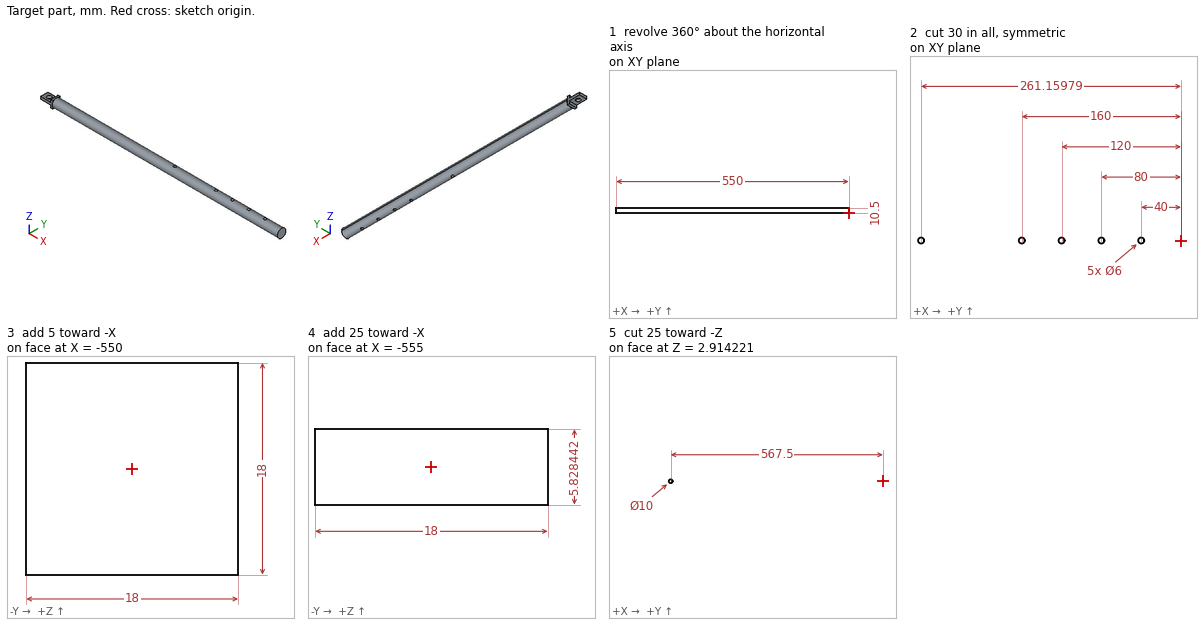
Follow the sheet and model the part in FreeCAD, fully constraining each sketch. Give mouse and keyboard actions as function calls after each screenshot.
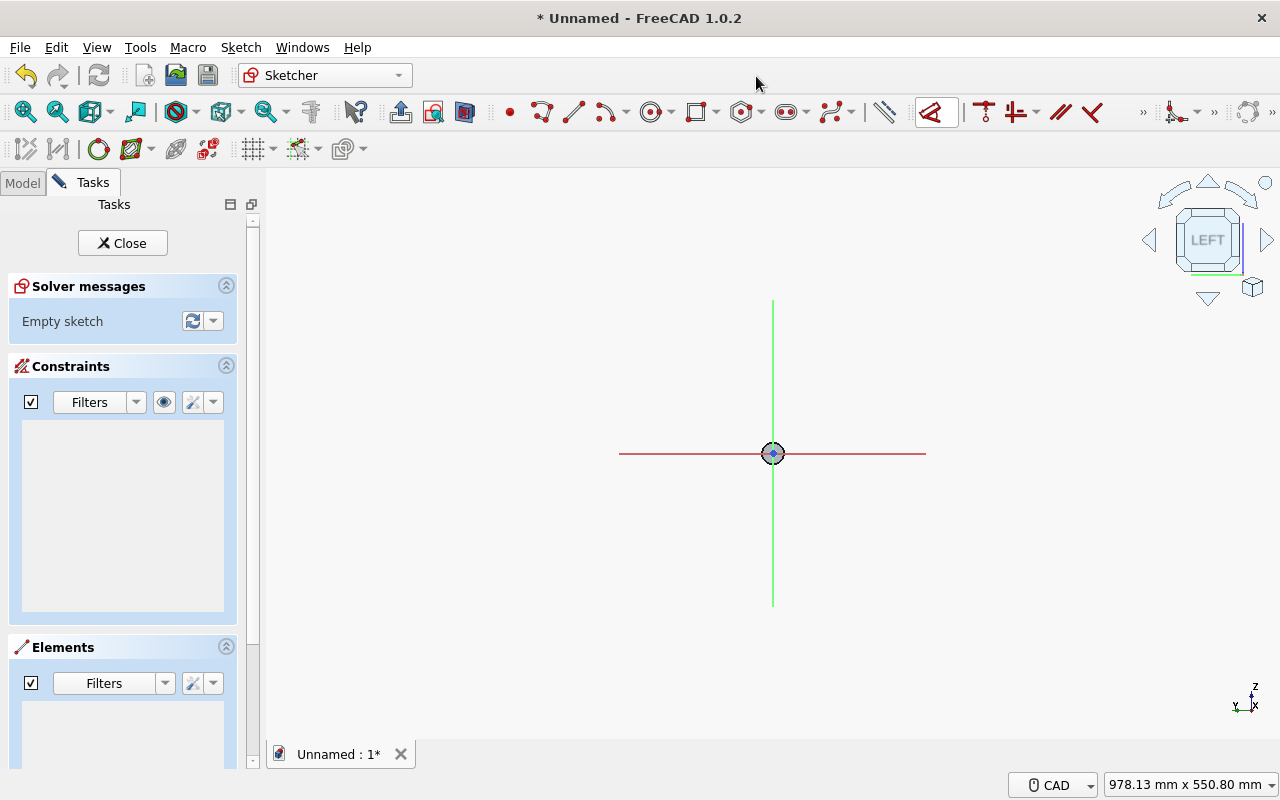
scroll(777, 454, up, 15)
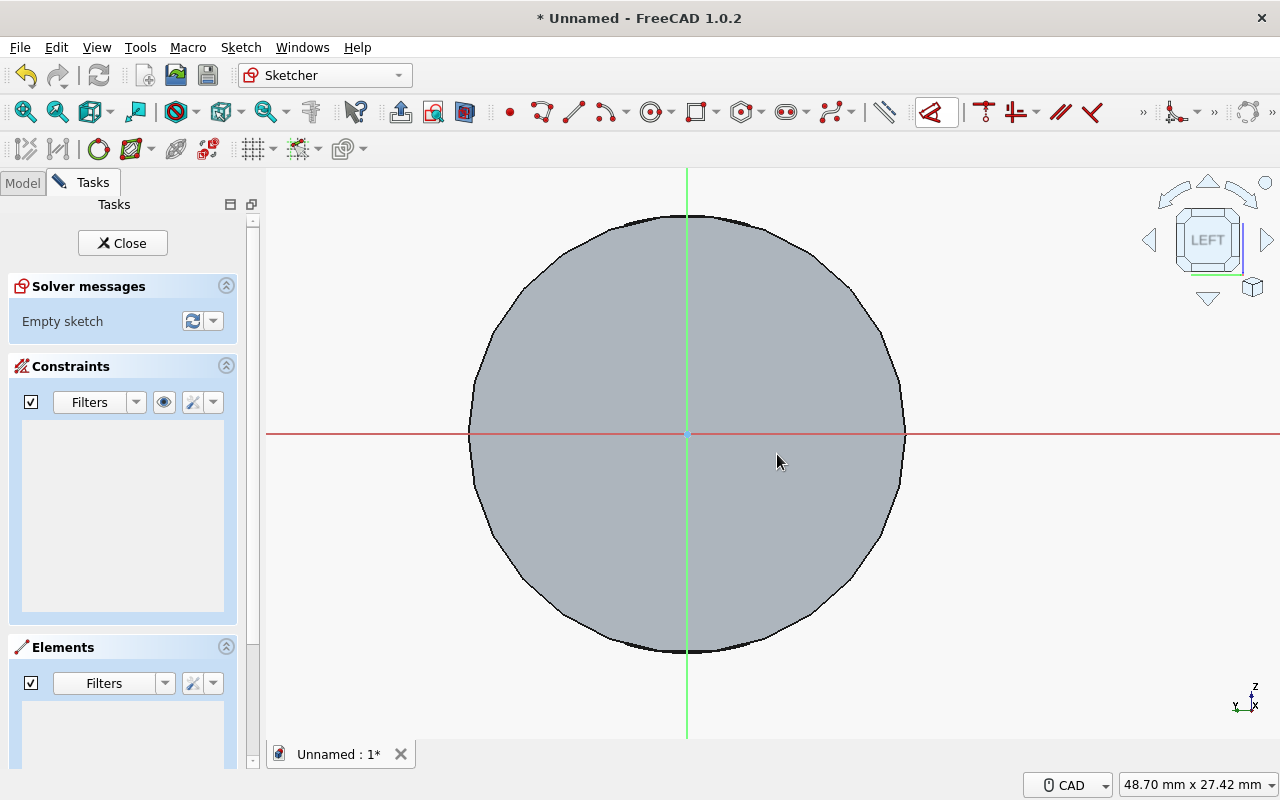
key(g)
key(v)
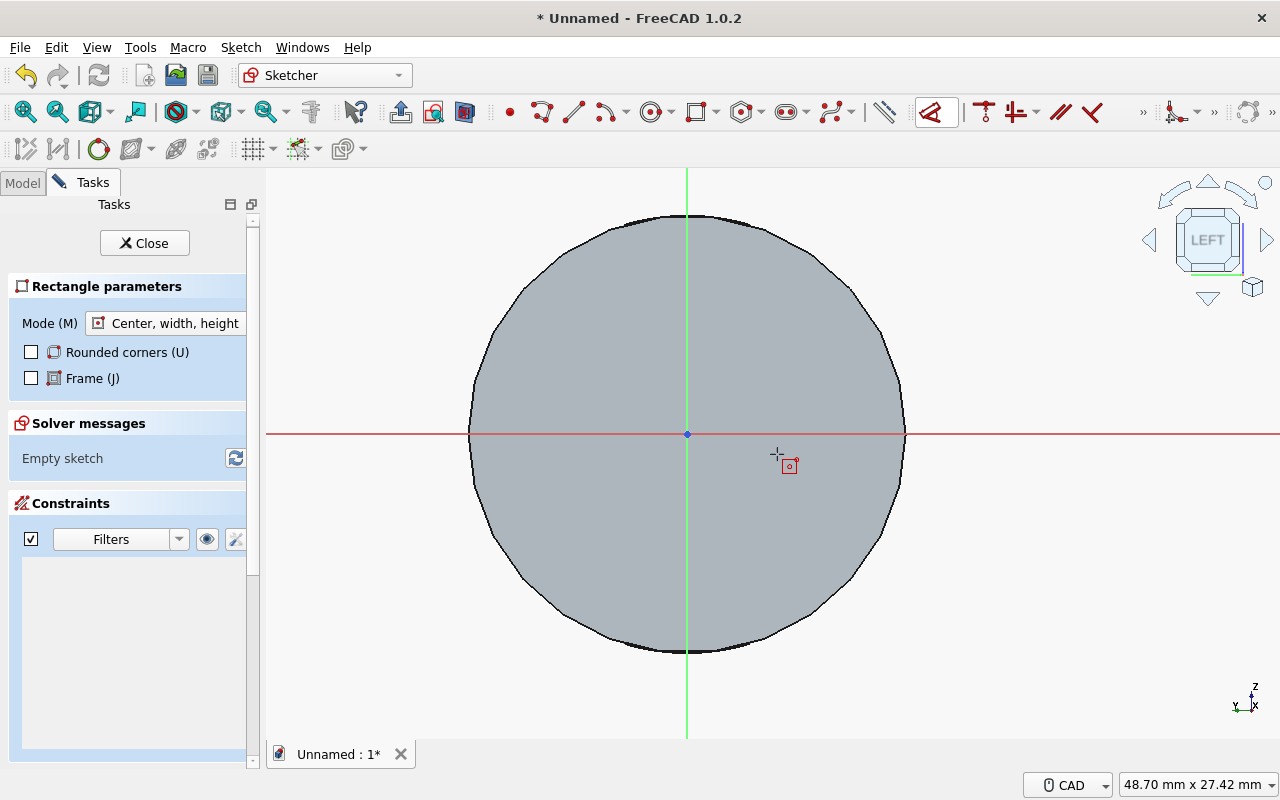
click(687, 434)
click(874, 247)
key(Escape)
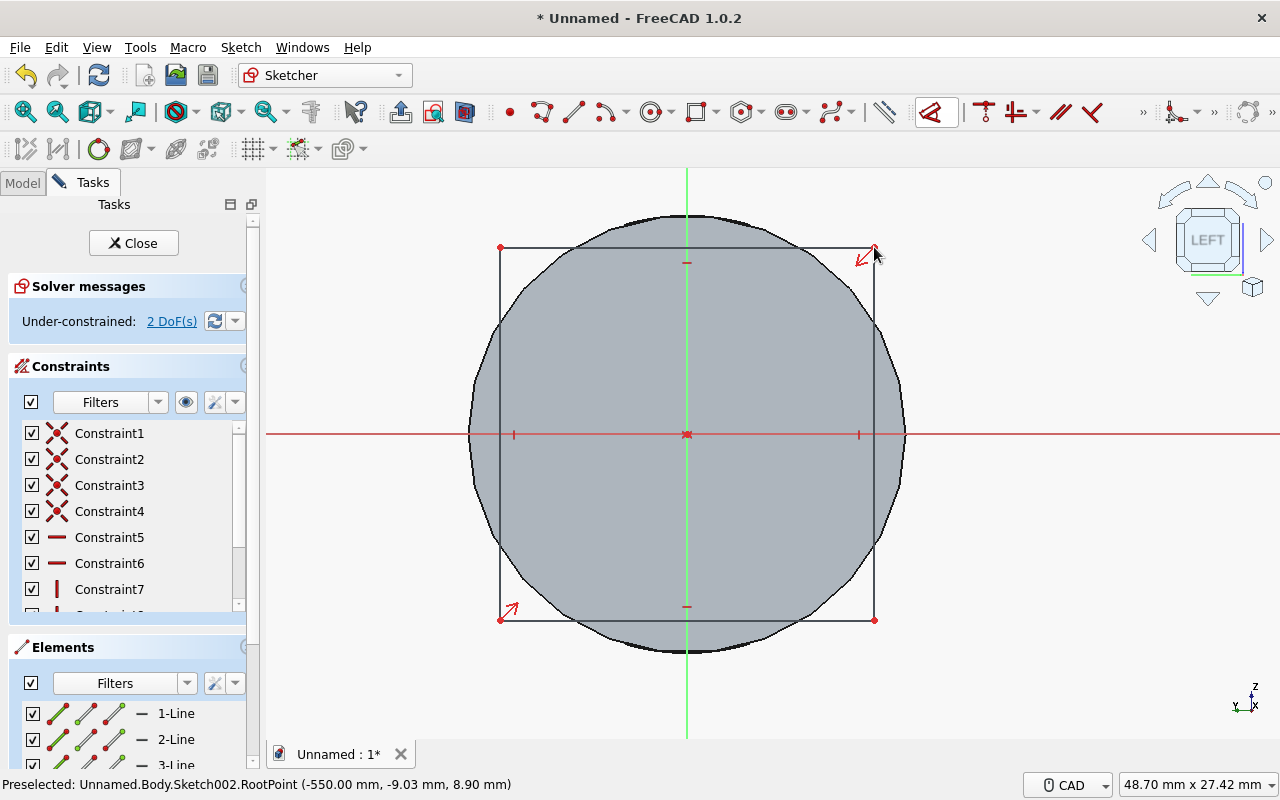
click(930, 112)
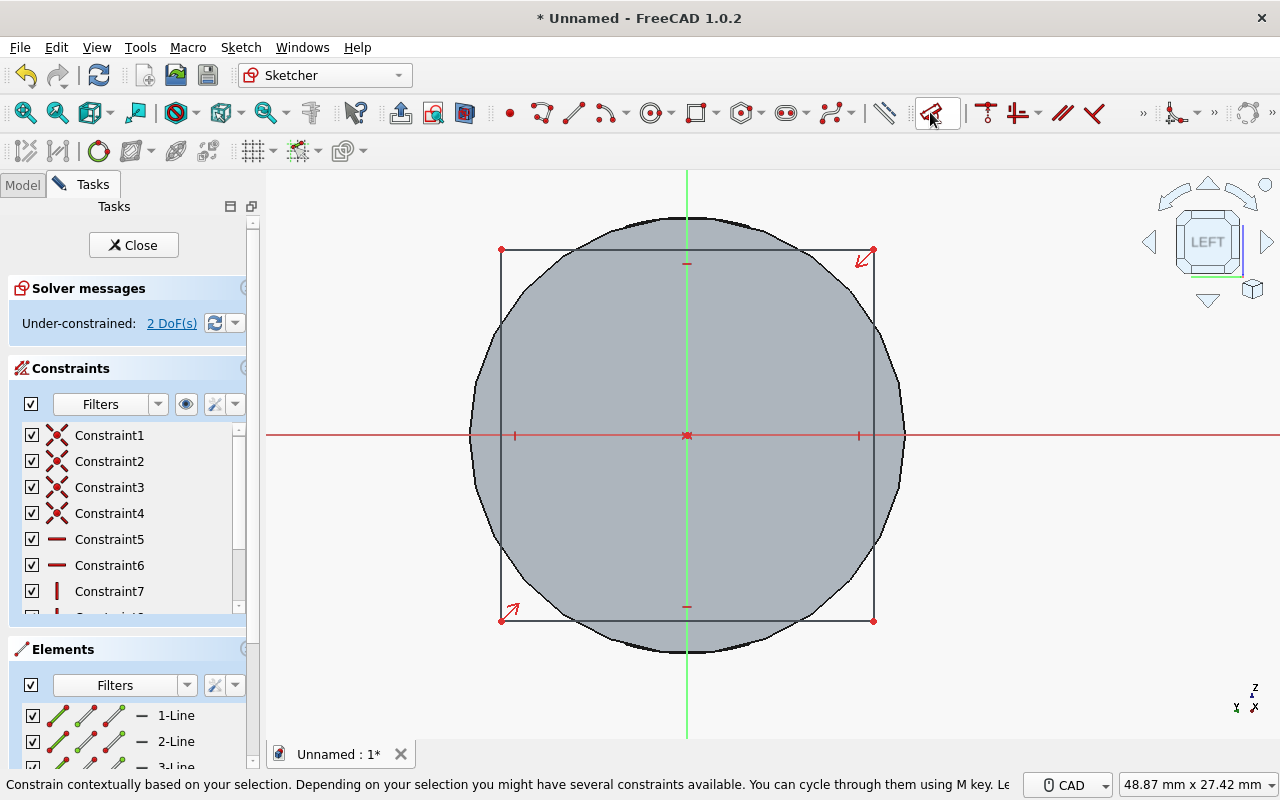
click(613, 621)
click(602, 655)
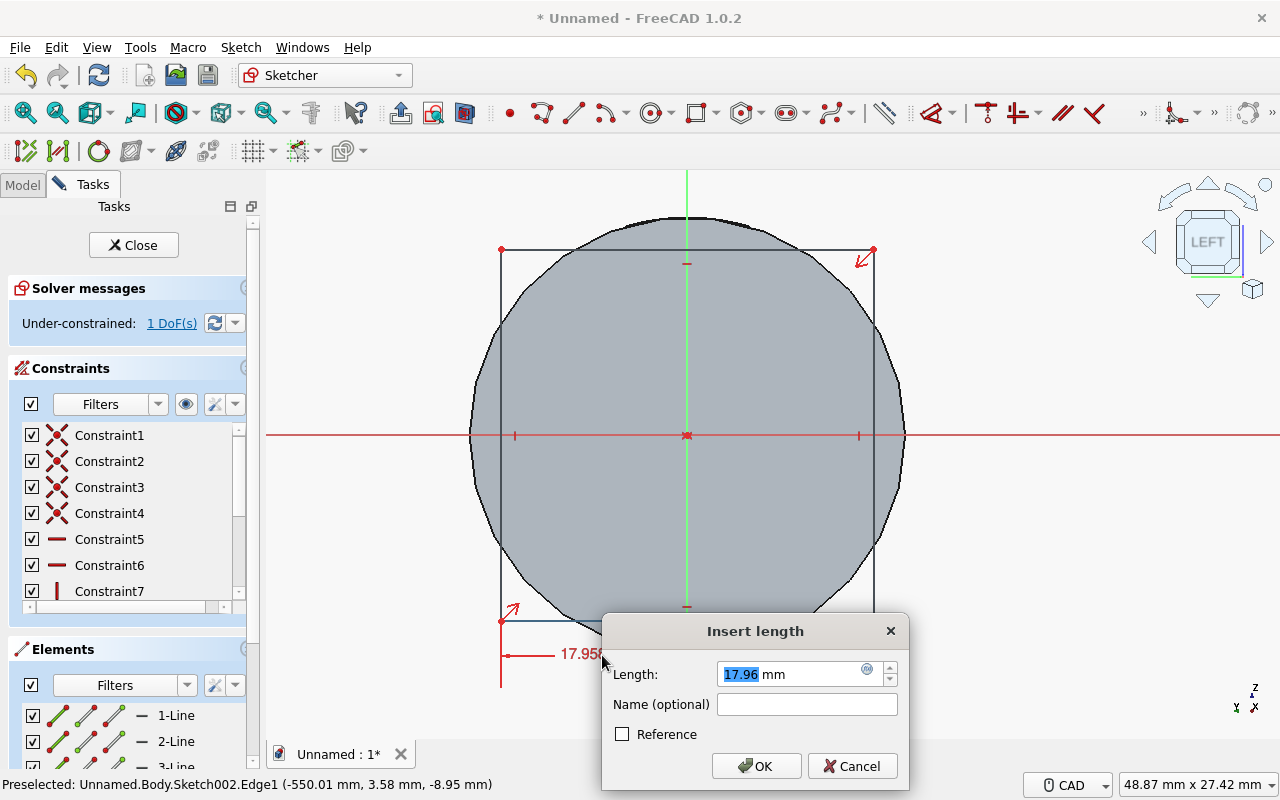
text(18)
key(Return)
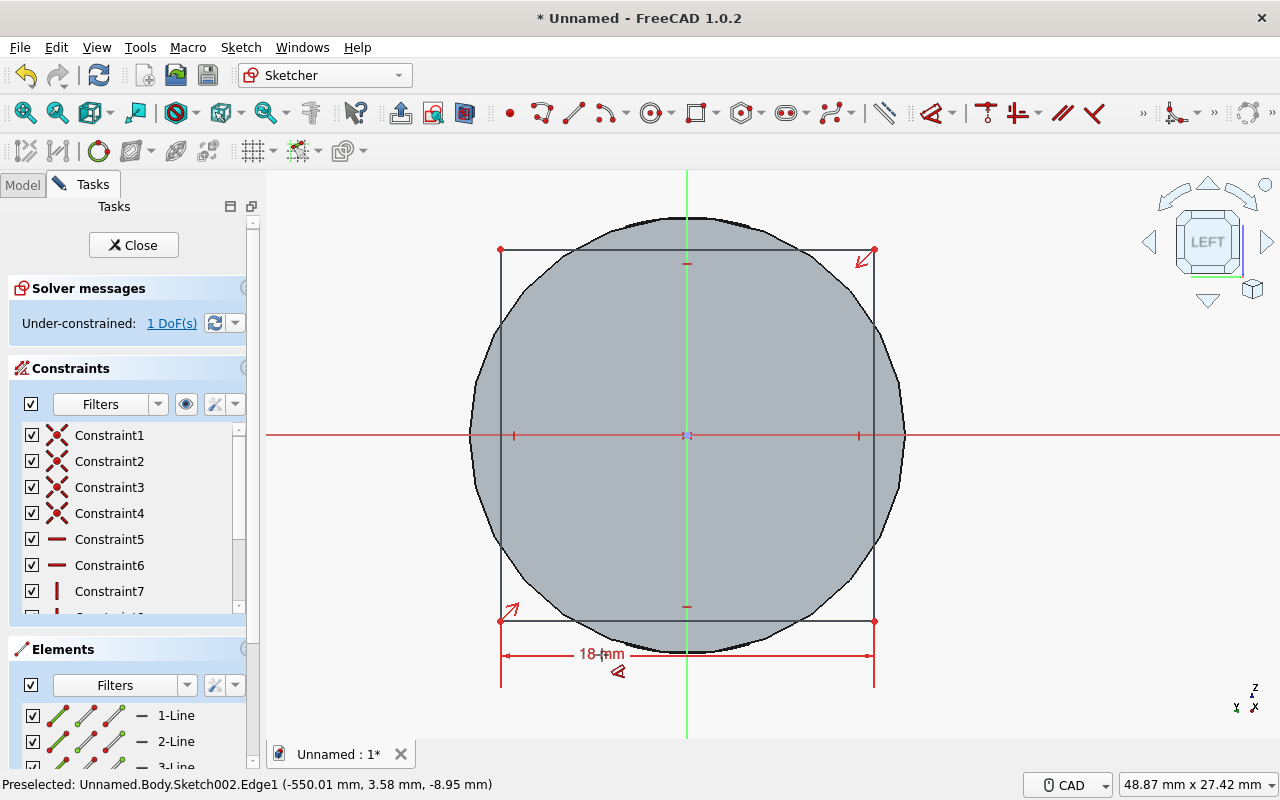
click(874, 510)
click(908, 350)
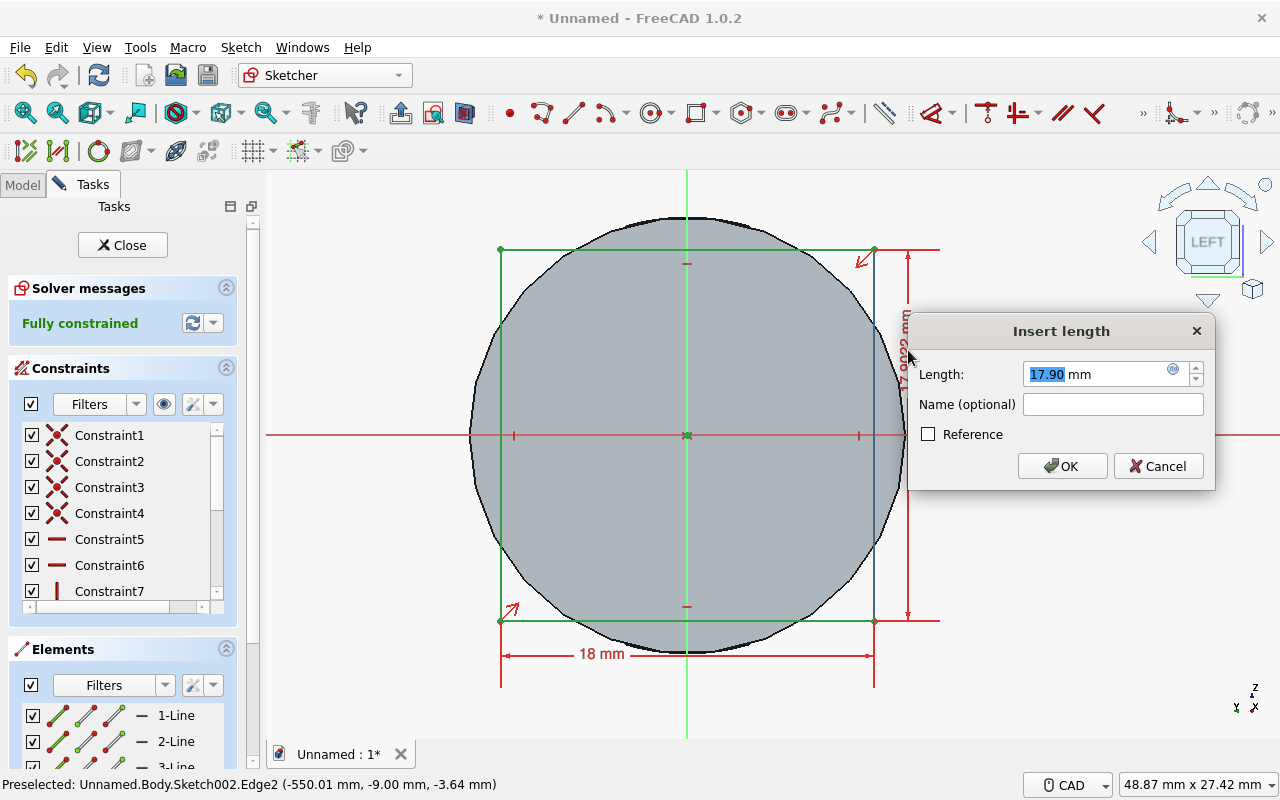
text(18)
key(Return)
key(Escape)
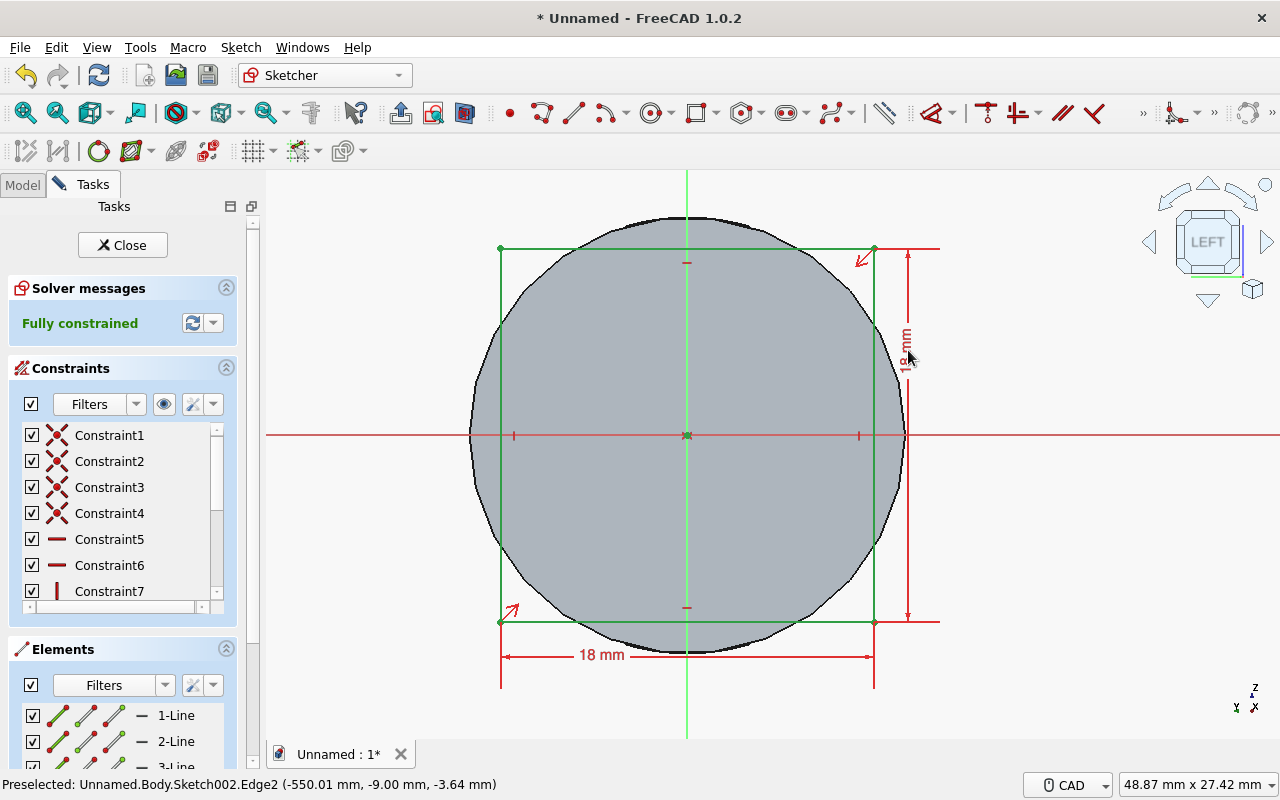
click(123, 245)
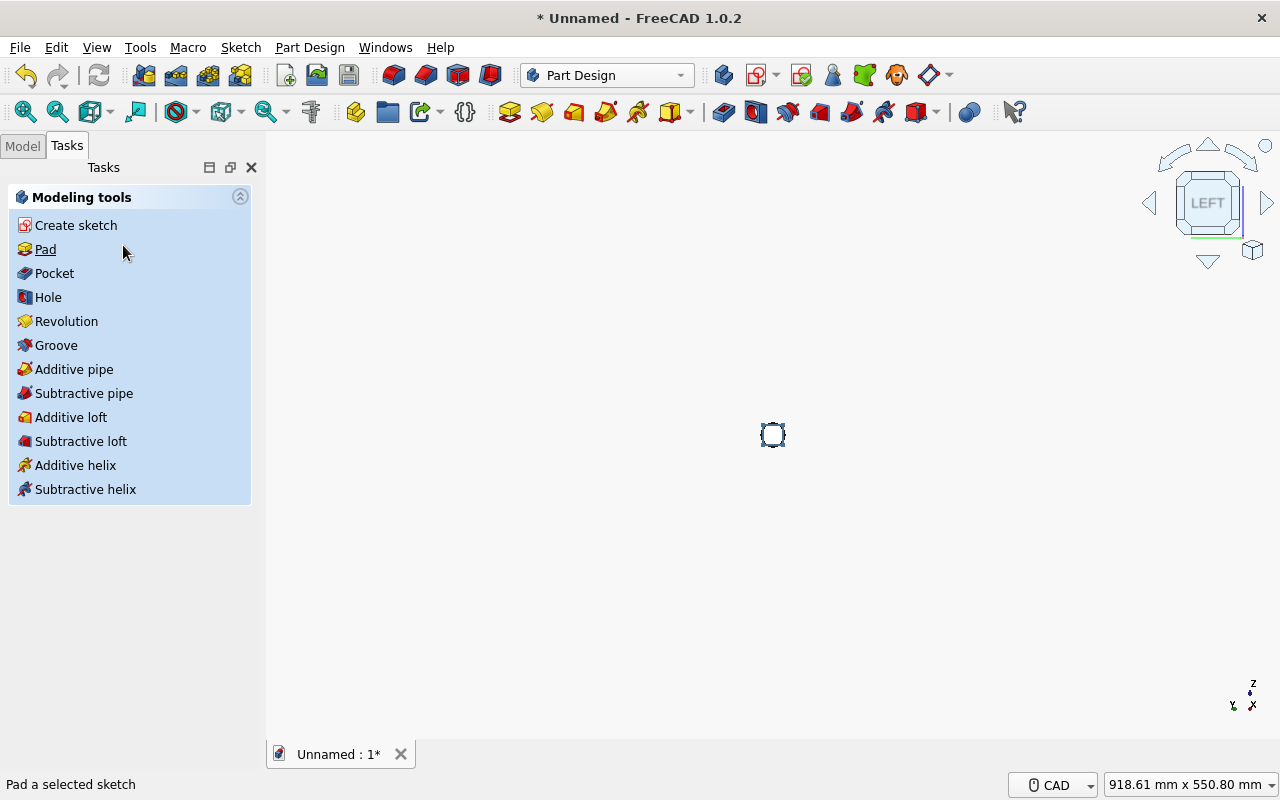
click(510, 112)